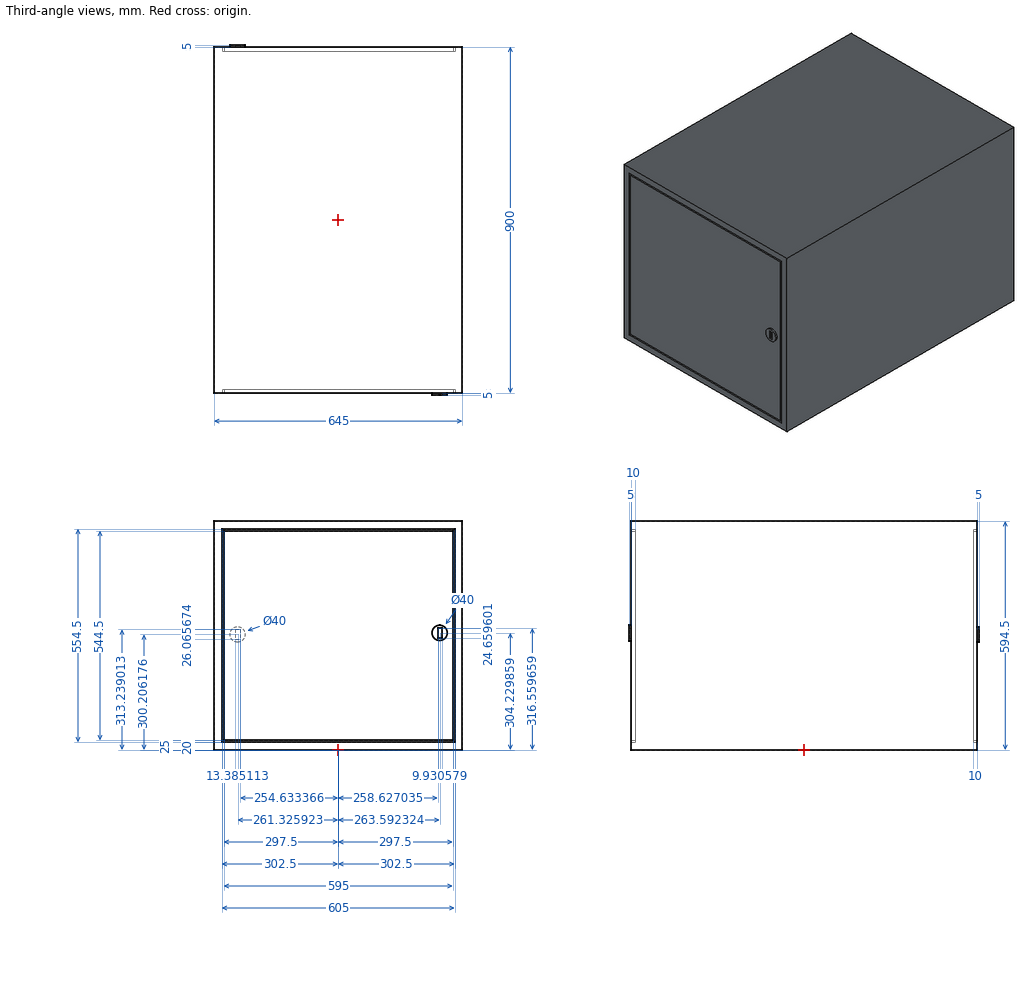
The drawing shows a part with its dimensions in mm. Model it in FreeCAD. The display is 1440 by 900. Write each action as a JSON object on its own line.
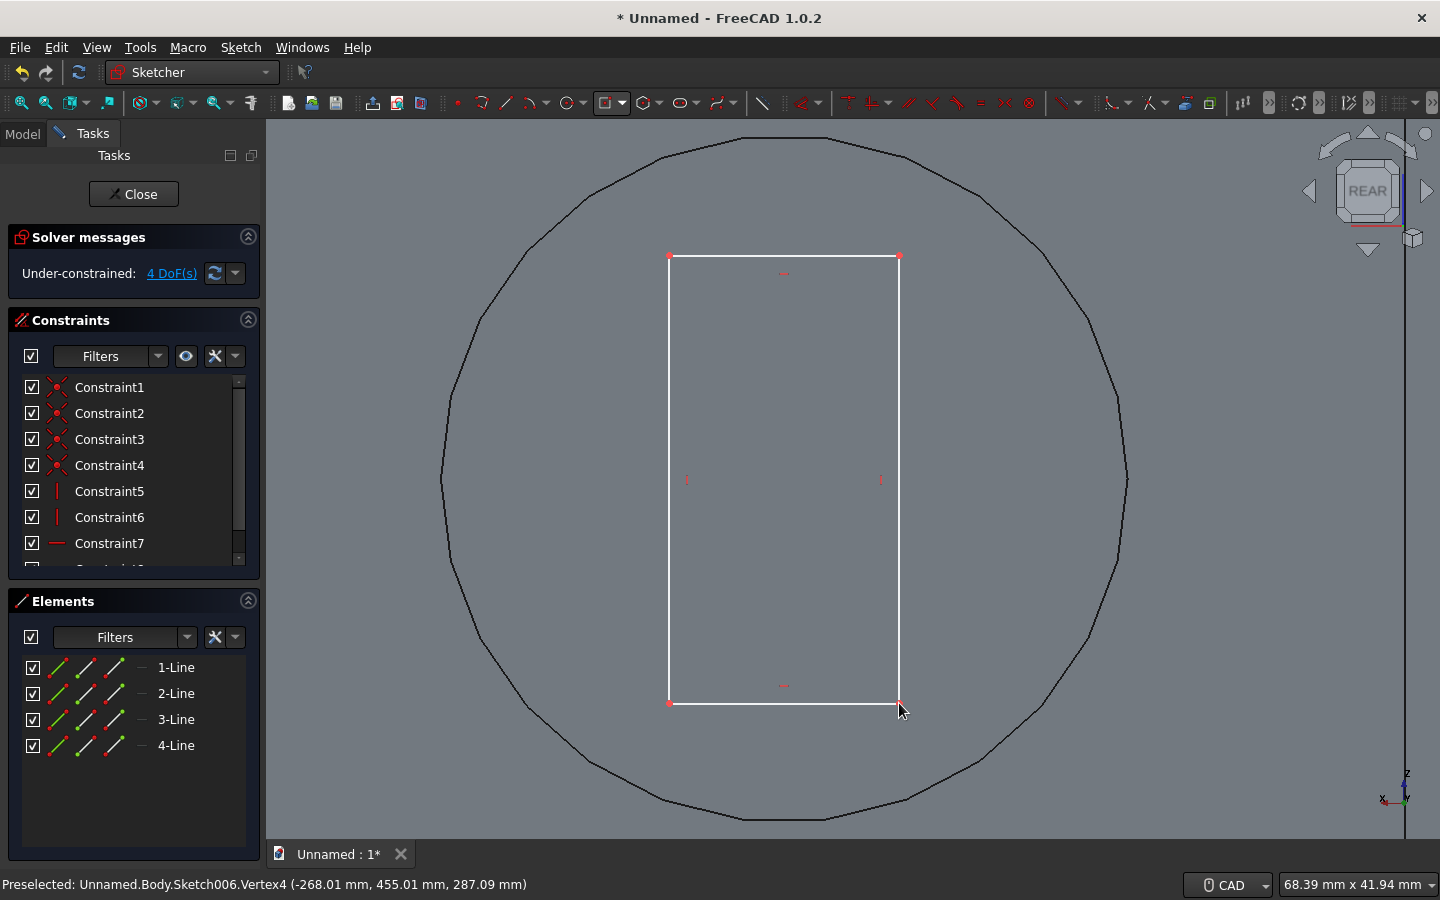
{"action": "left_click", "coordinate": [802, 104]}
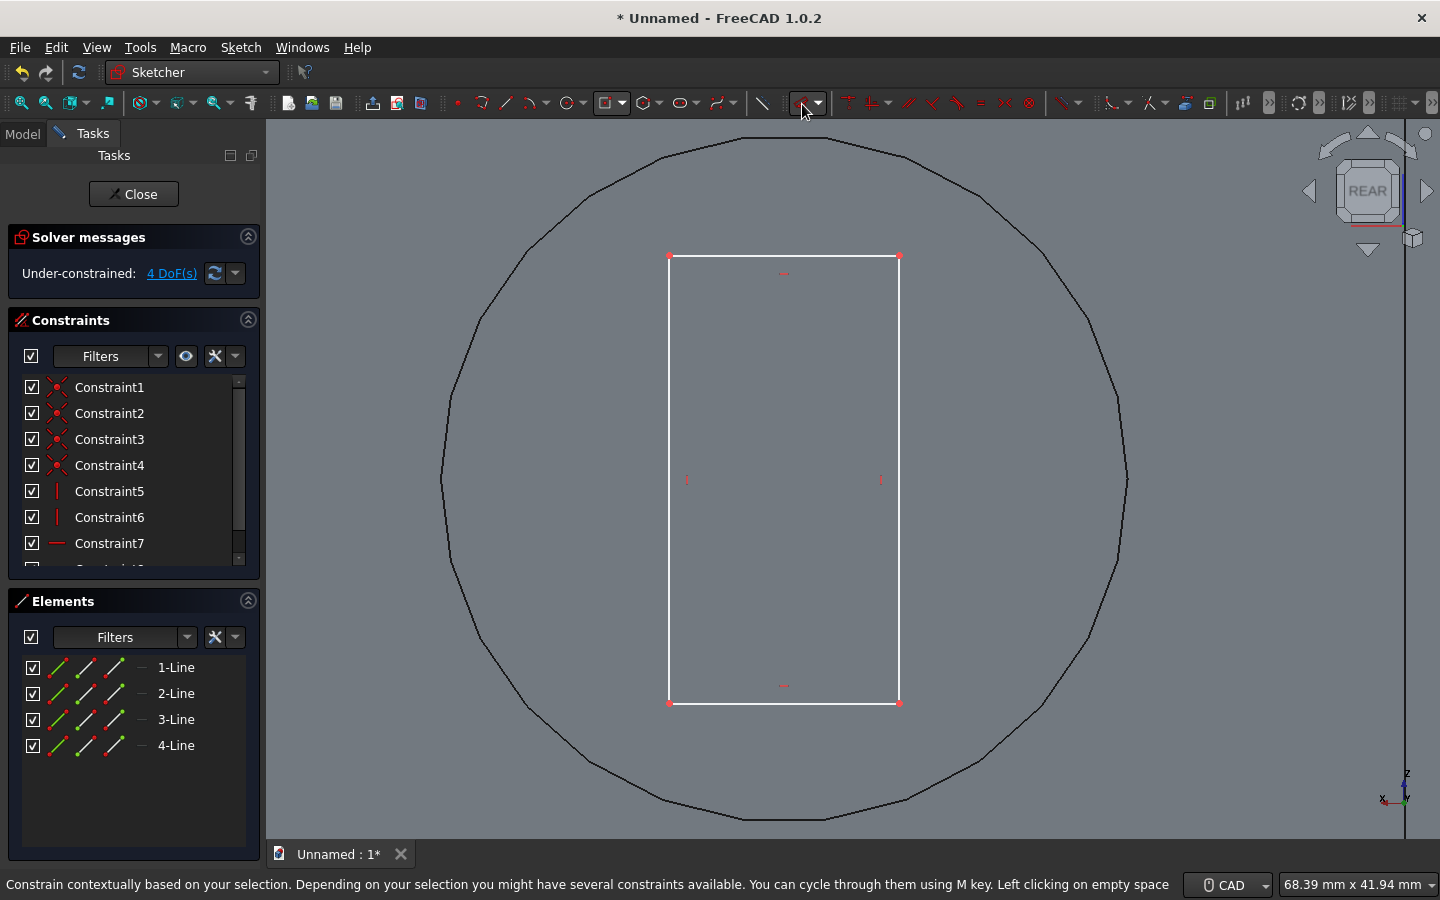
{"action": "left_click", "coordinate": [669, 390]}
{"action": "left_click", "coordinate": [635, 480]}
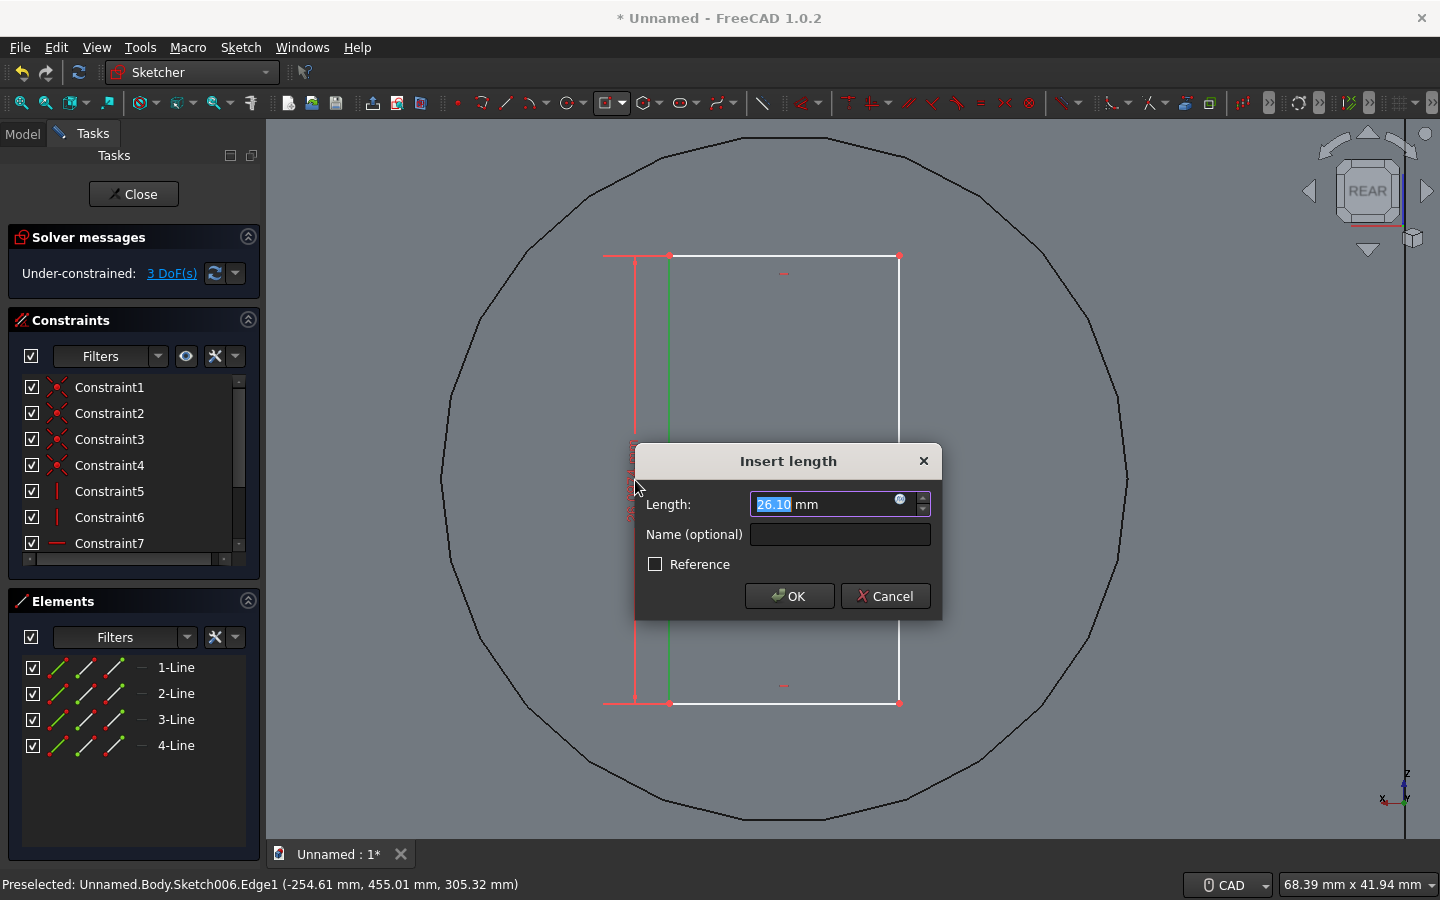
{"action": "type", "text": "26.065674"}
{"action": "key", "text": "Return"}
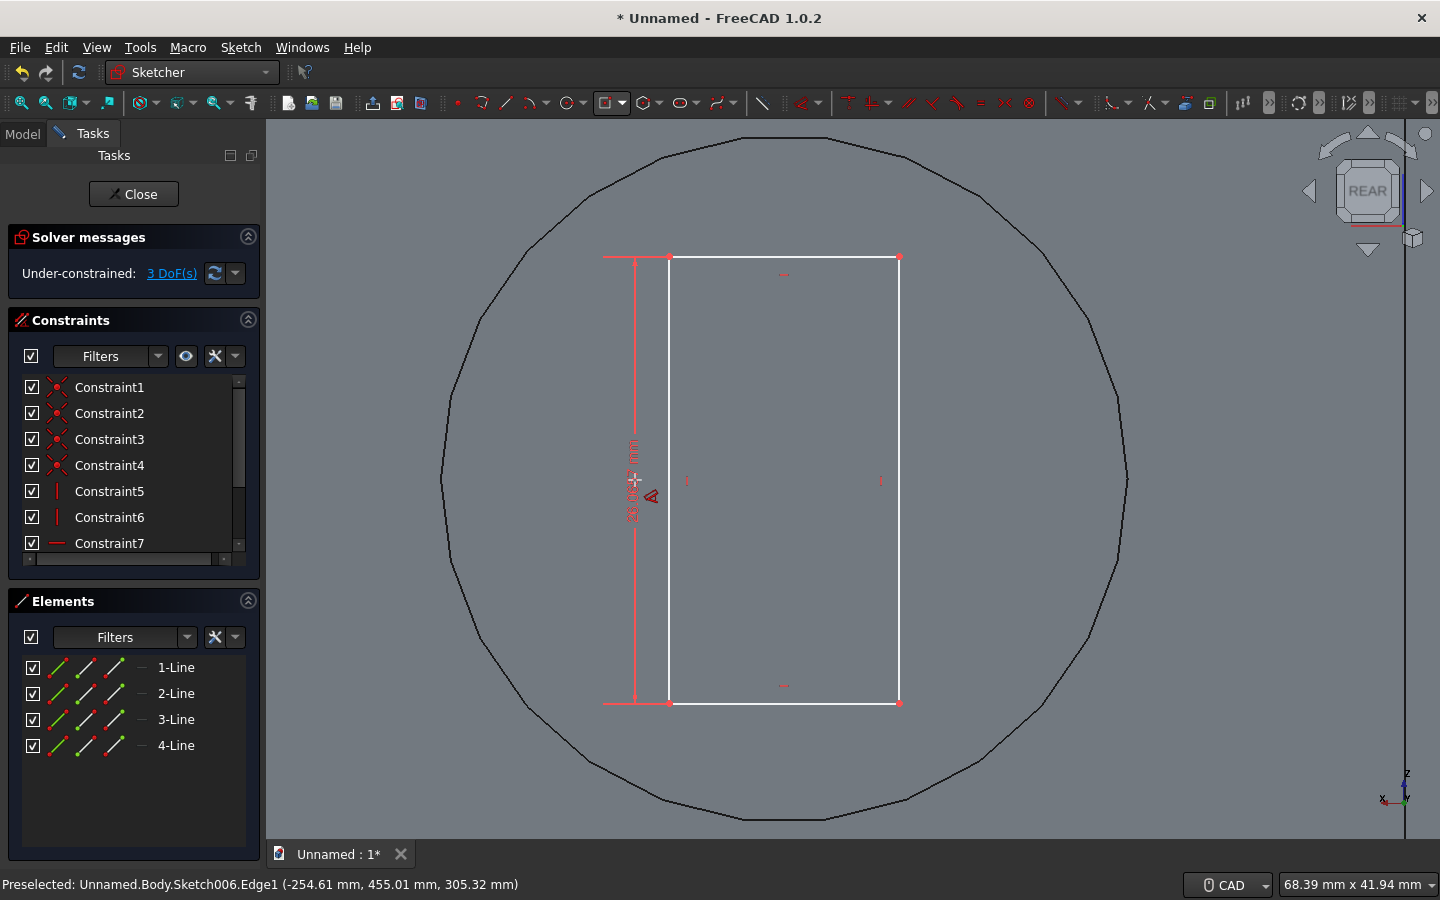
{"action": "left_click", "coordinate": [738, 704]}
{"action": "left_click", "coordinate": [784, 738]}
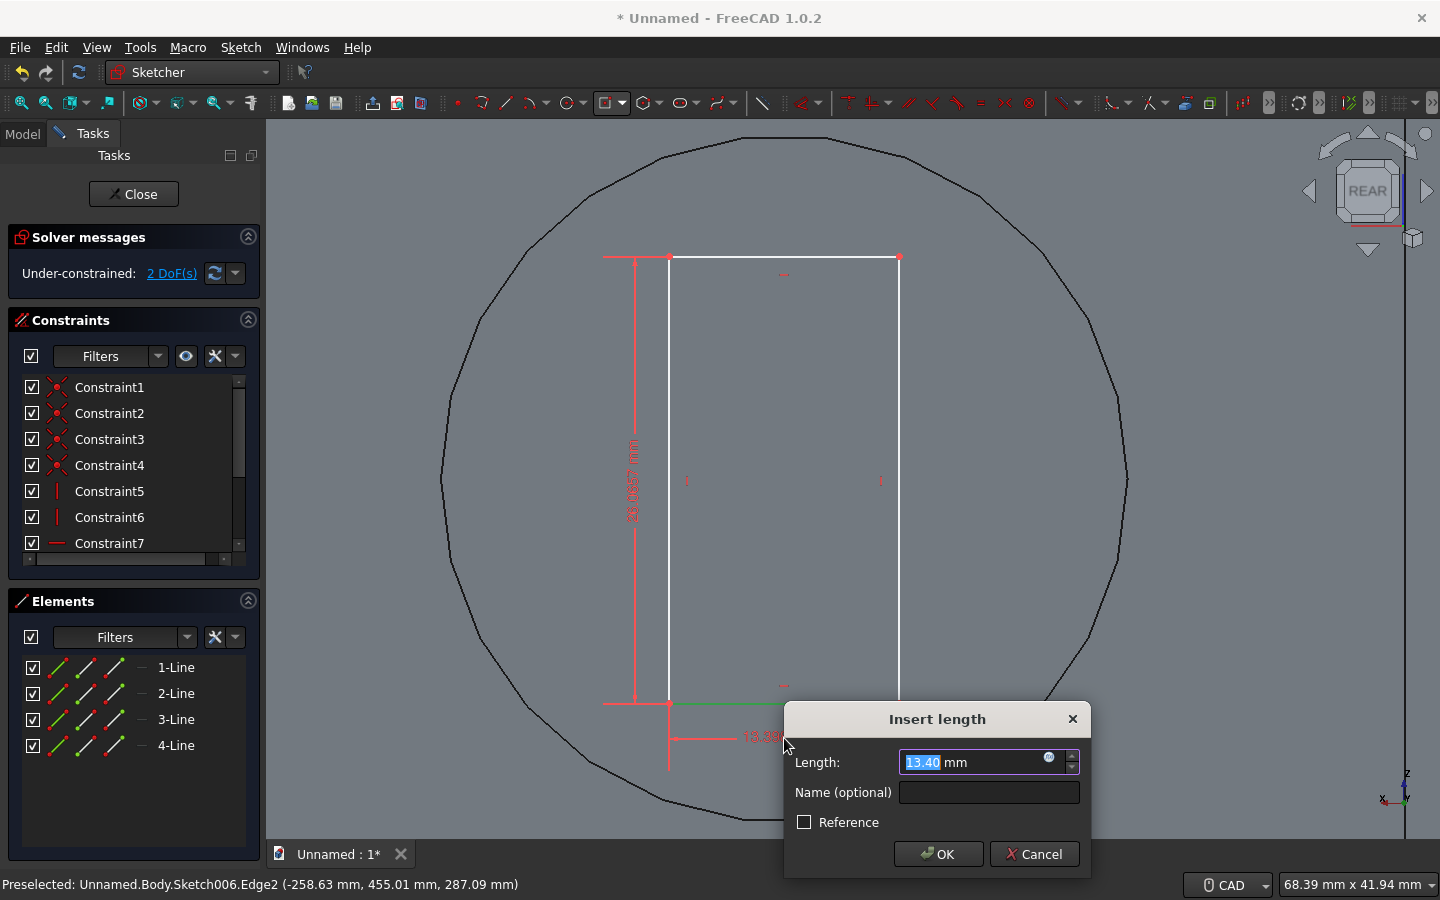
{"action": "type", "text": "13.385113"}
{"action": "key", "text": "Return"}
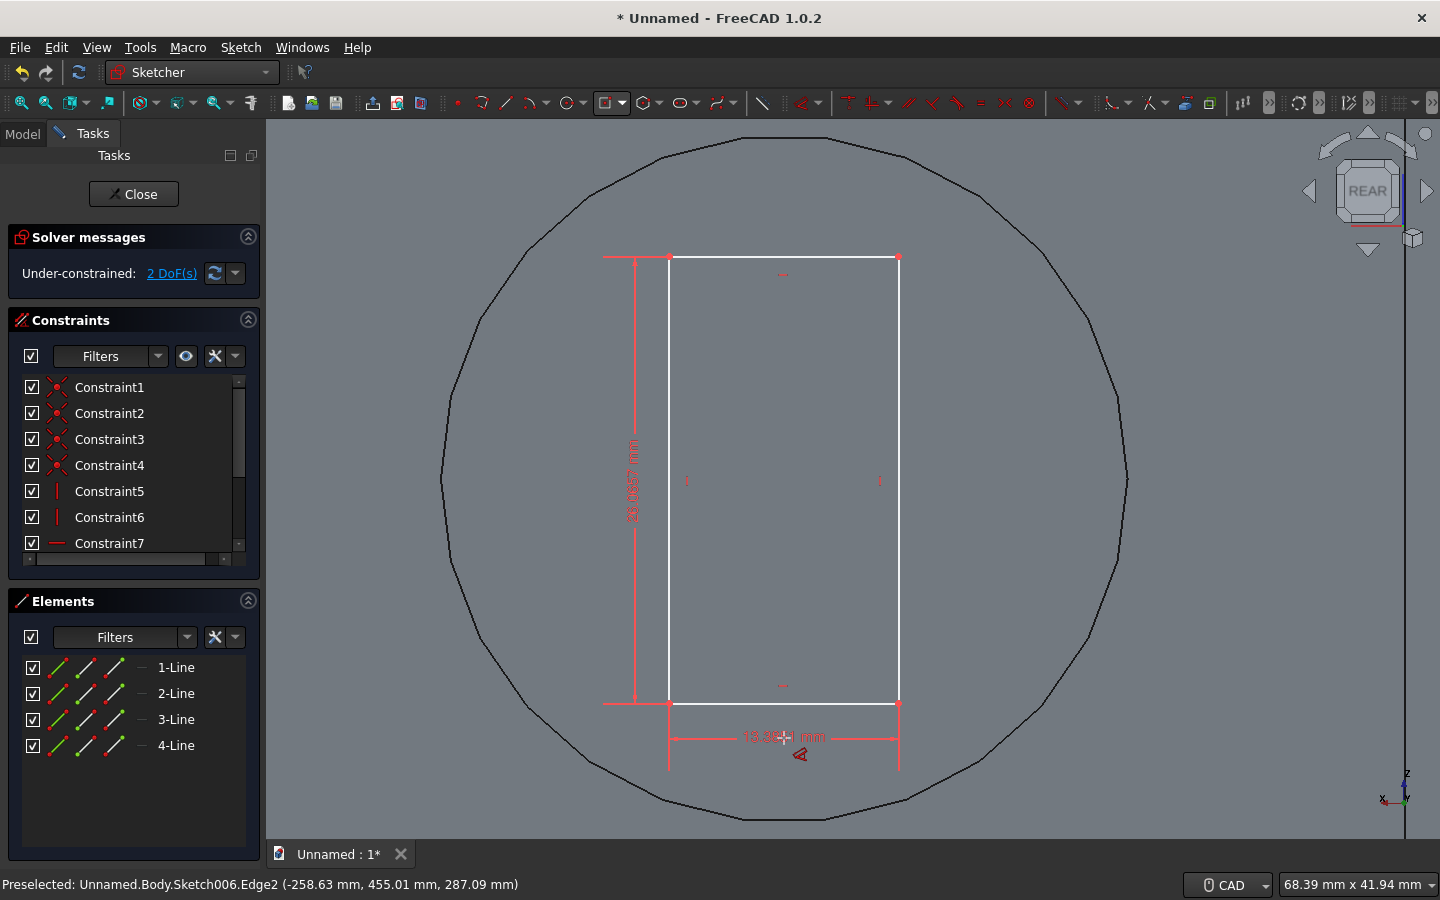
{"action": "left_click", "coordinate": [669, 257]}
{"action": "left_click", "coordinate": [481, 223]}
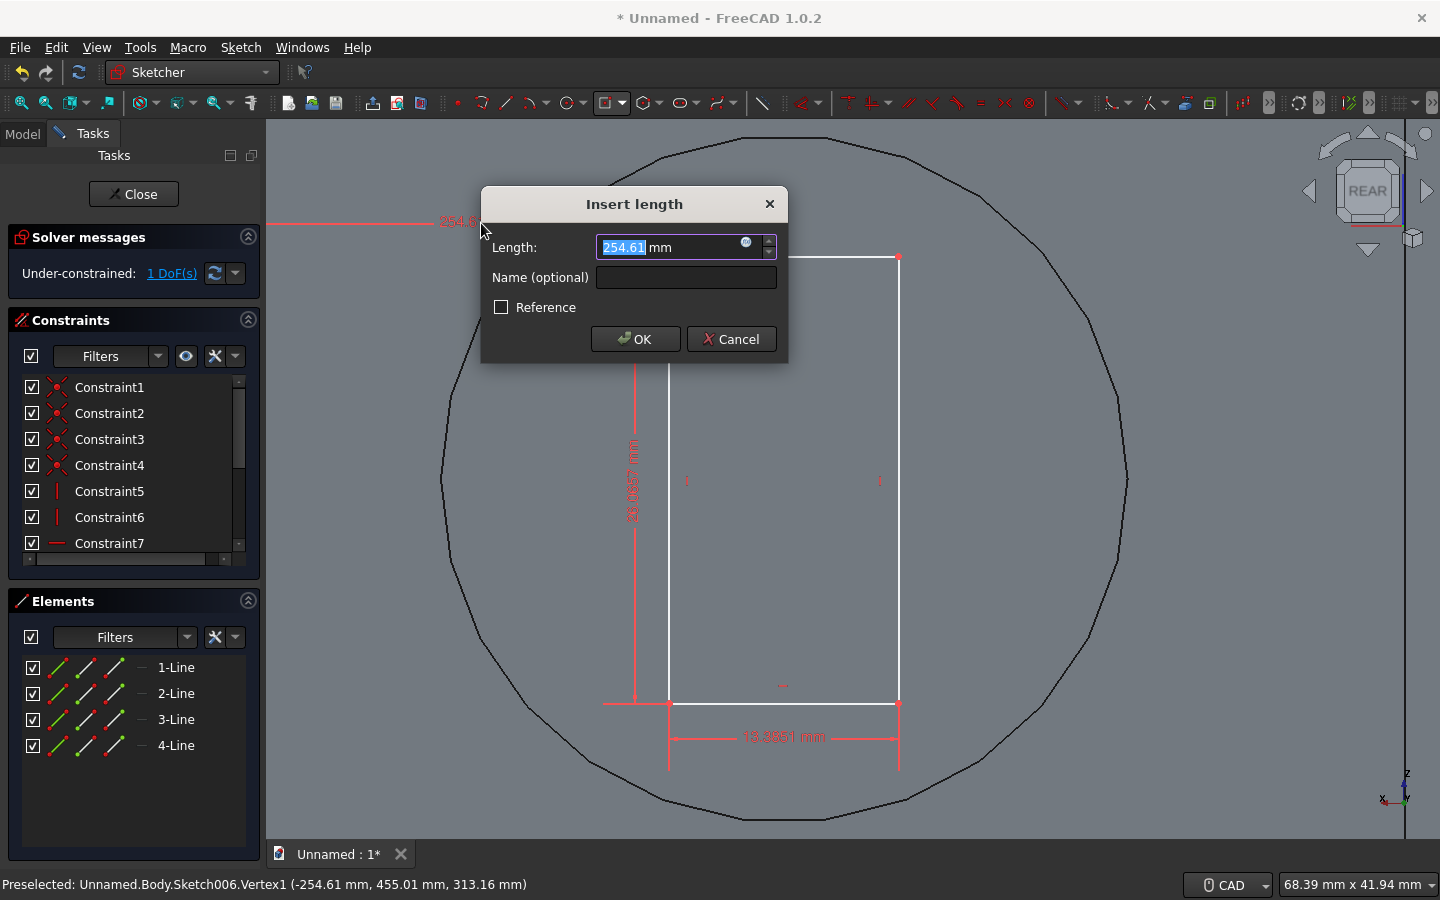
{"action": "type", "text": "254.633366"}
{"action": "key", "text": "Return"}